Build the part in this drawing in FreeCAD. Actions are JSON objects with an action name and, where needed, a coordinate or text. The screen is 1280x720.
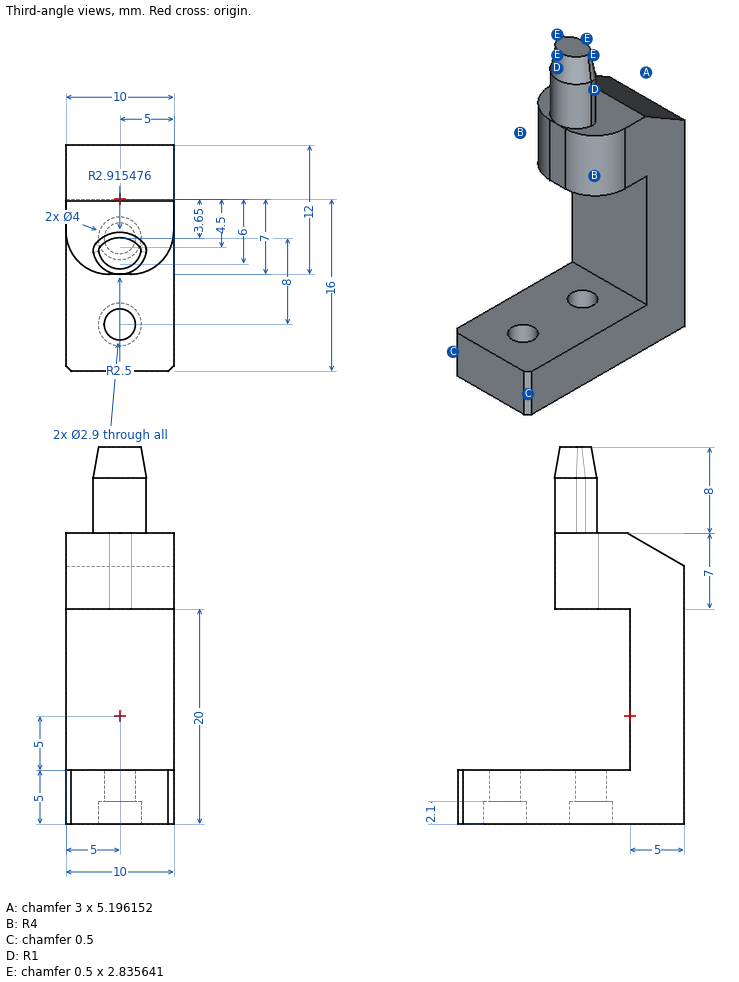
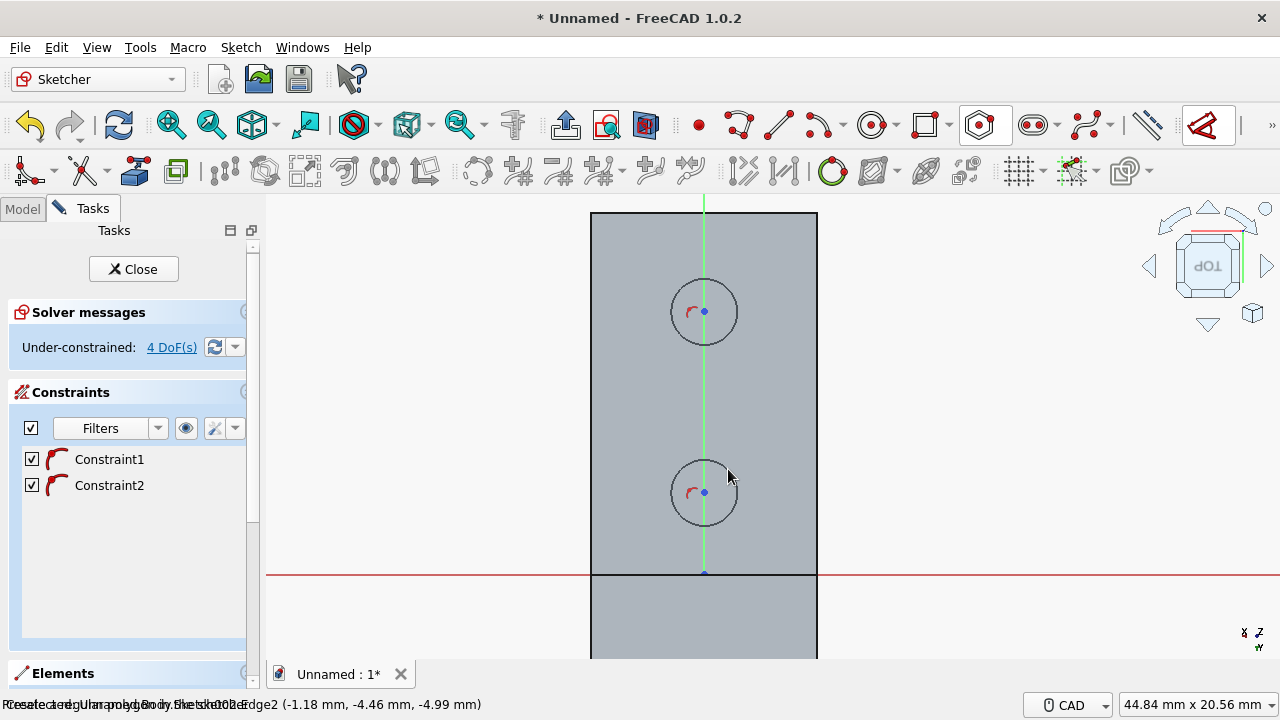
{"action": "left_click", "coordinate": [728, 289]}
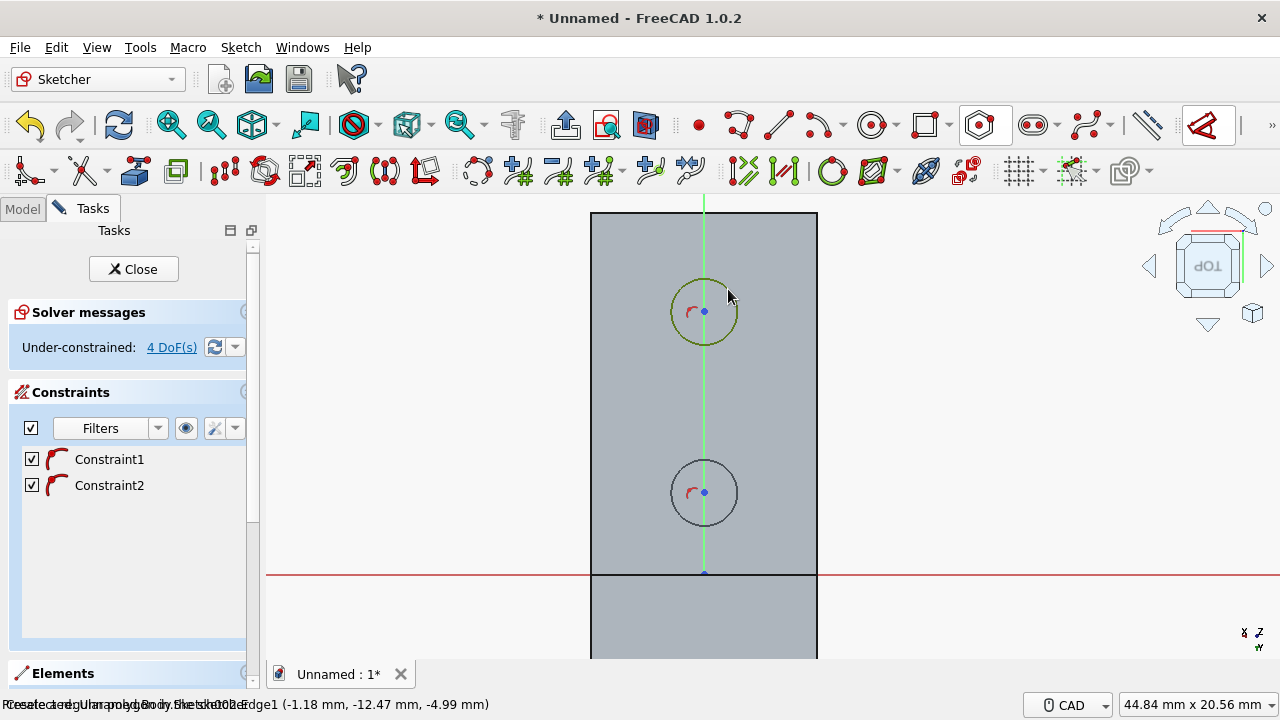
{"action": "left_click", "coordinate": [728, 470]}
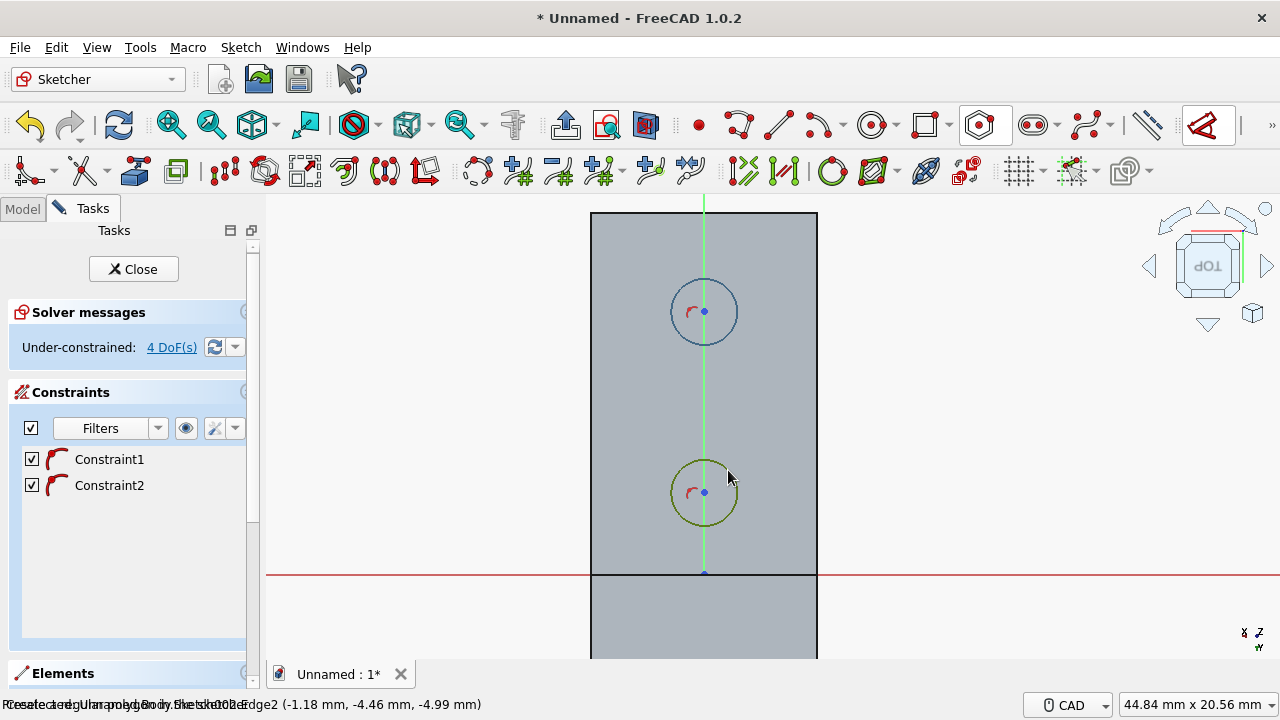
{"action": "key", "text": "e"}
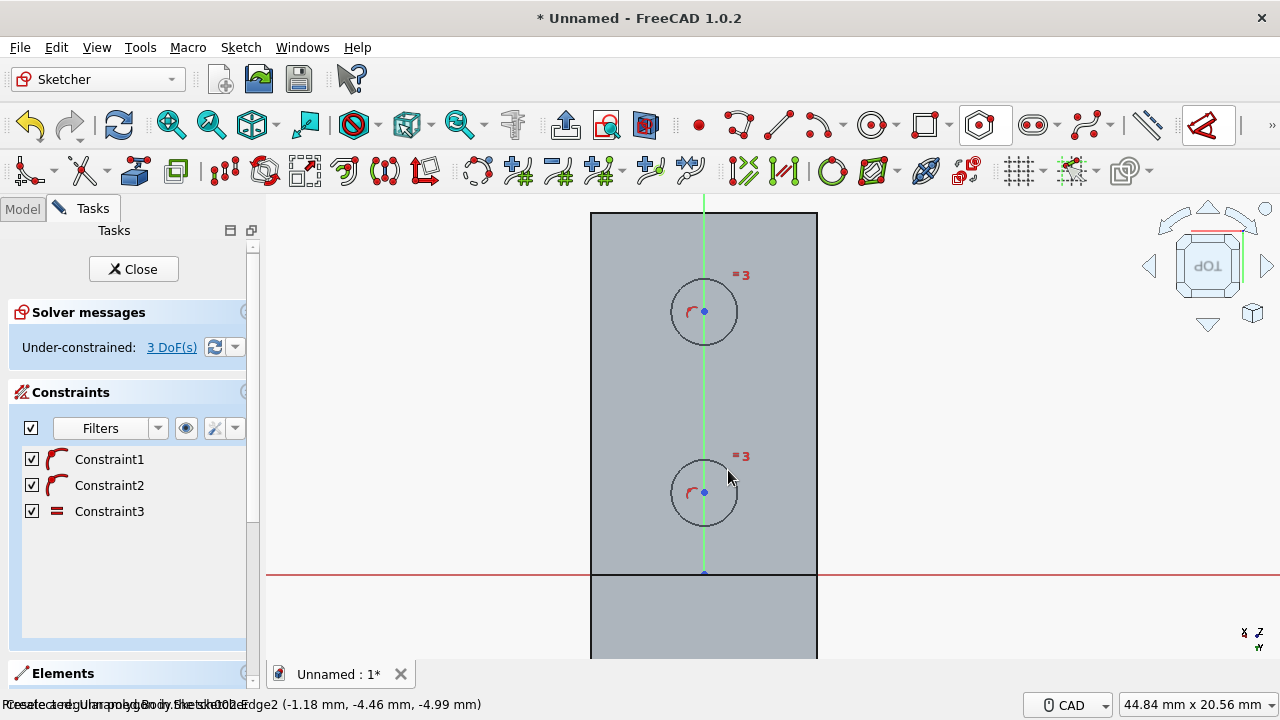
{"action": "key", "text": "d"}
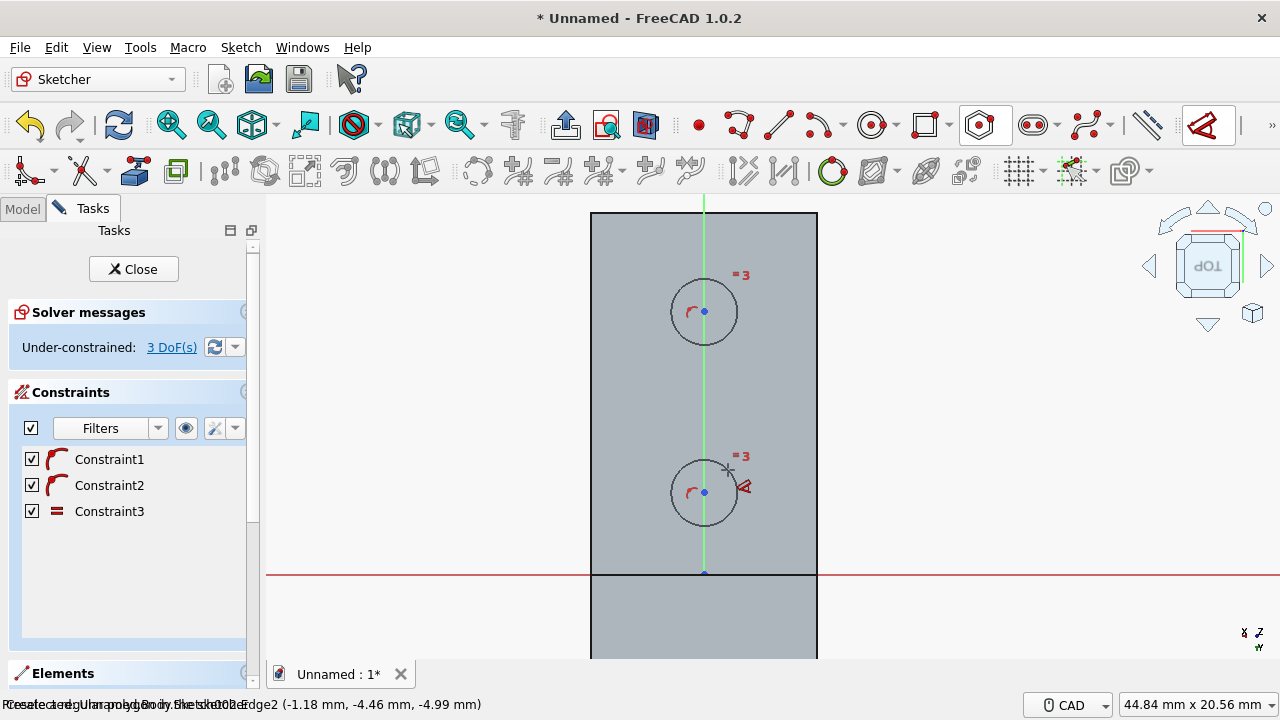
{"action": "left_click", "coordinate": [728, 289]}
{"action": "left_click", "coordinate": [751, 267]}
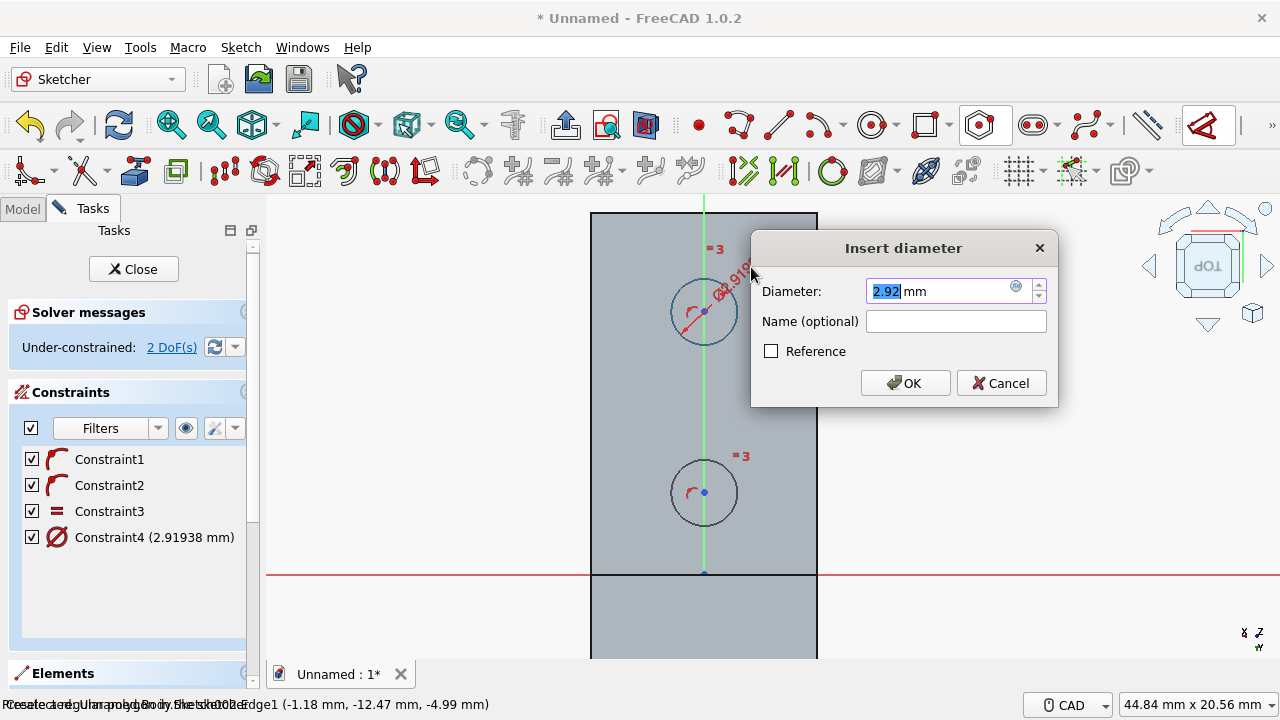
{"action": "type", "text": "2.9"}
{"action": "key", "text": "Return"}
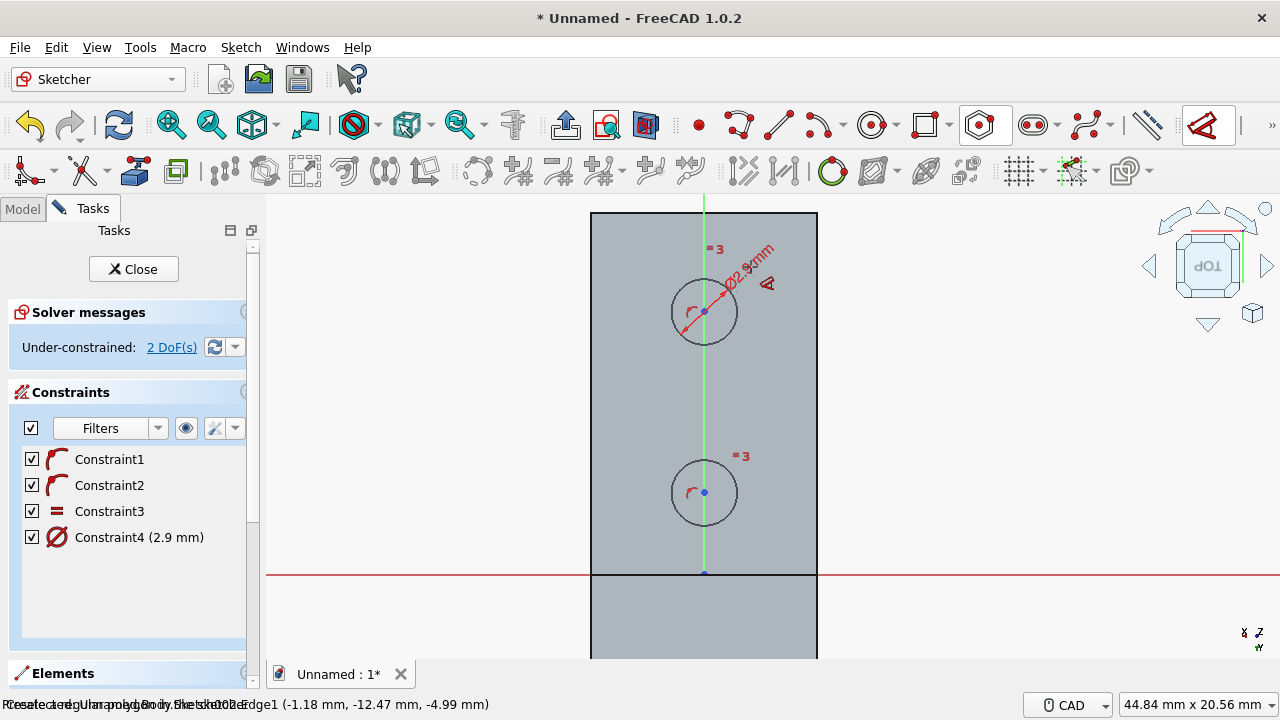
{"action": "left_click", "coordinate": [704, 312]}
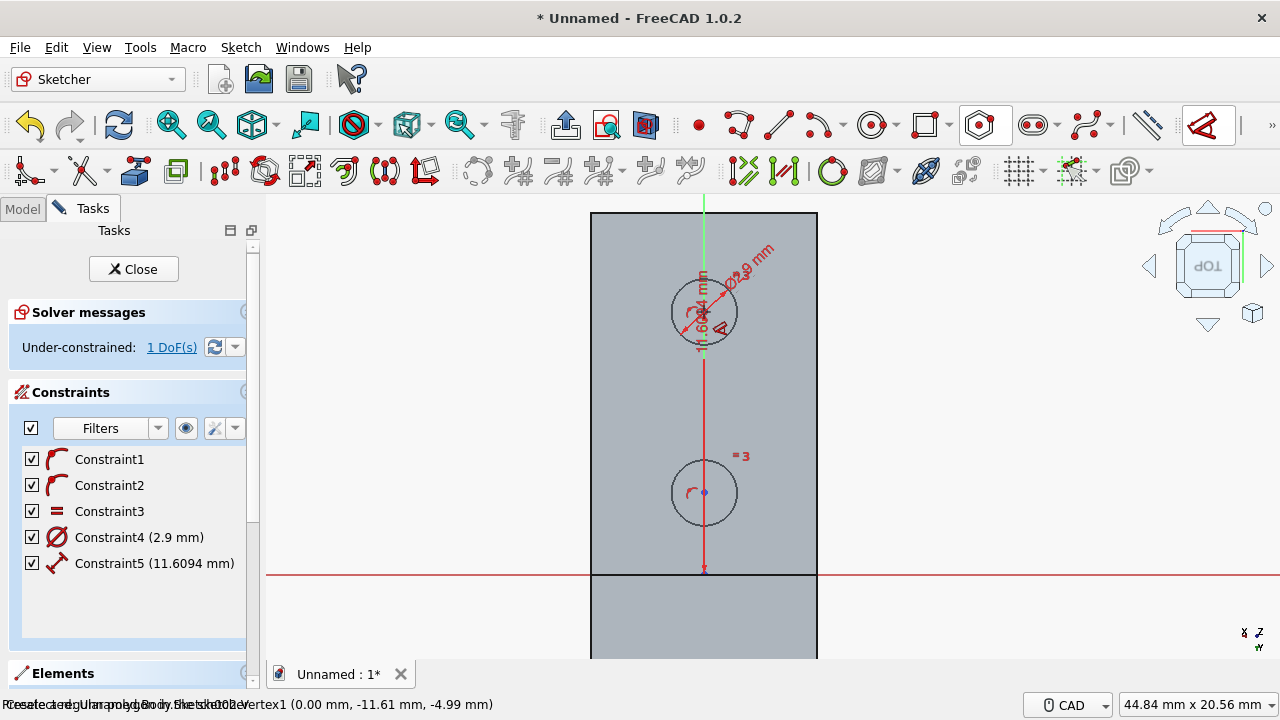
{"action": "left_click", "coordinate": [704, 493]}
{"action": "left_click", "coordinate": [738, 403]}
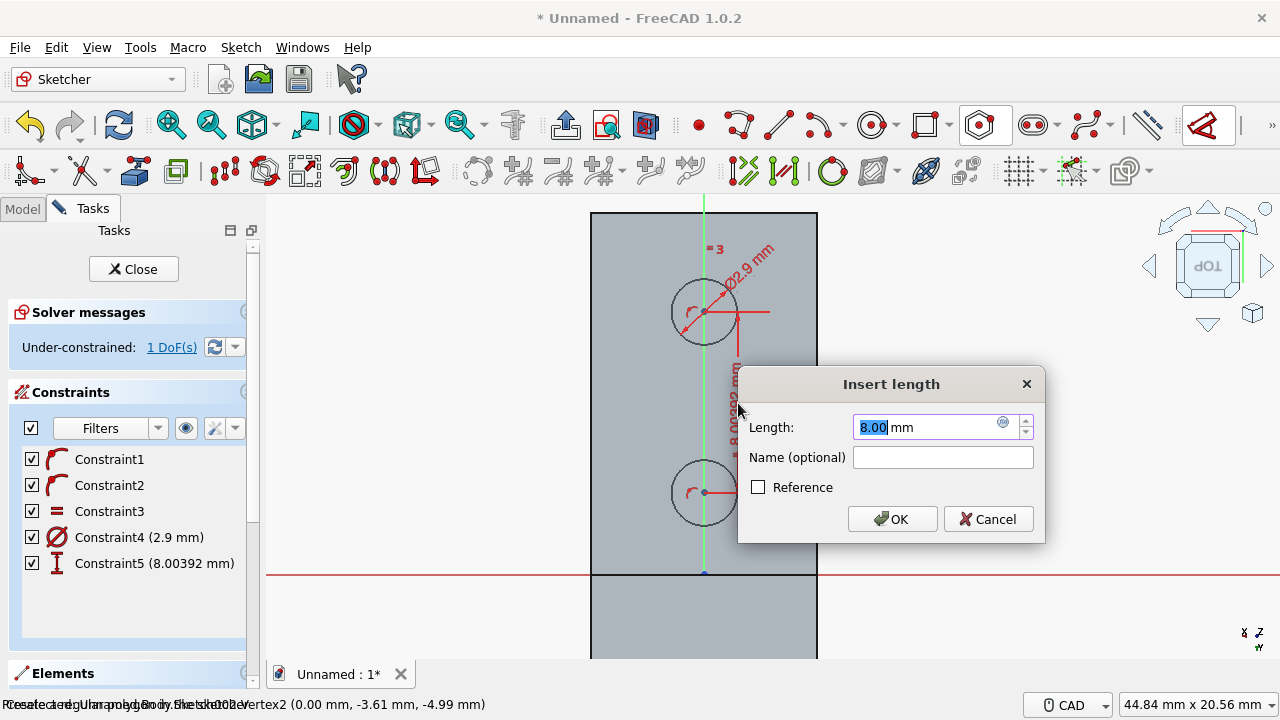
{"action": "type", "text": "8"}
{"action": "key", "text": "Return"}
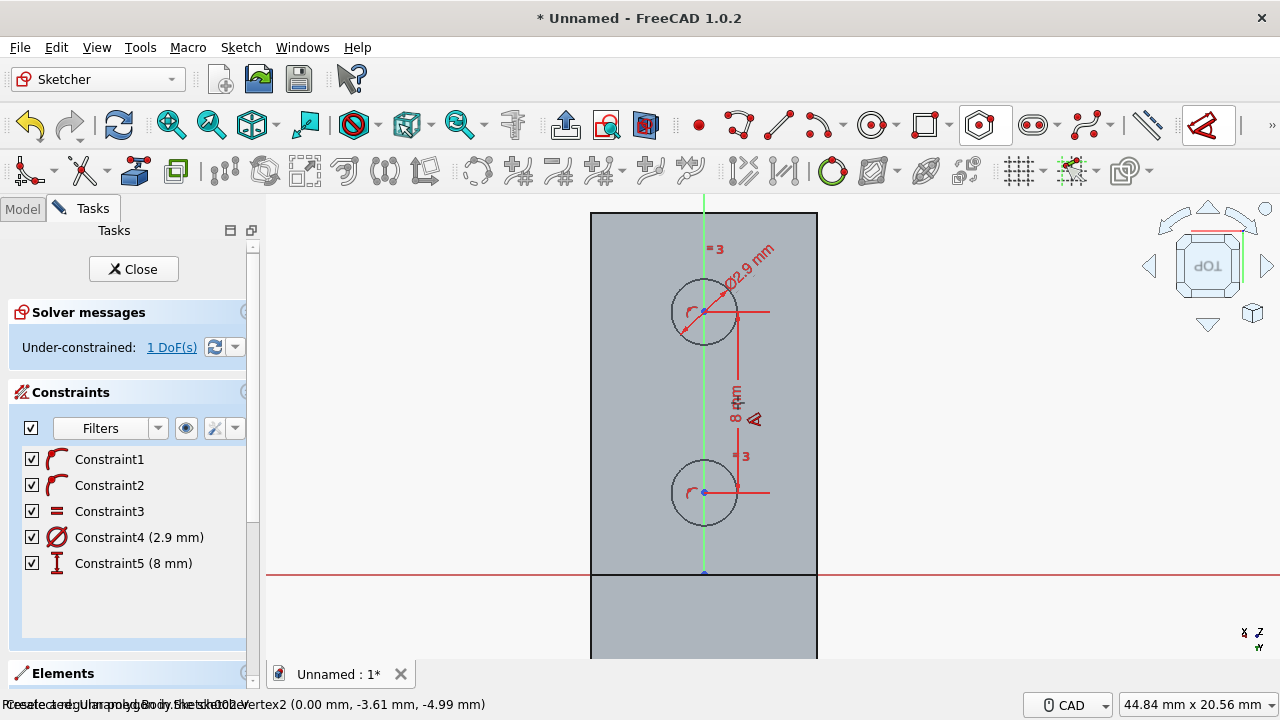
{"action": "left_click", "coordinate": [704, 493]}
{"action": "left_click", "coordinate": [738, 534]}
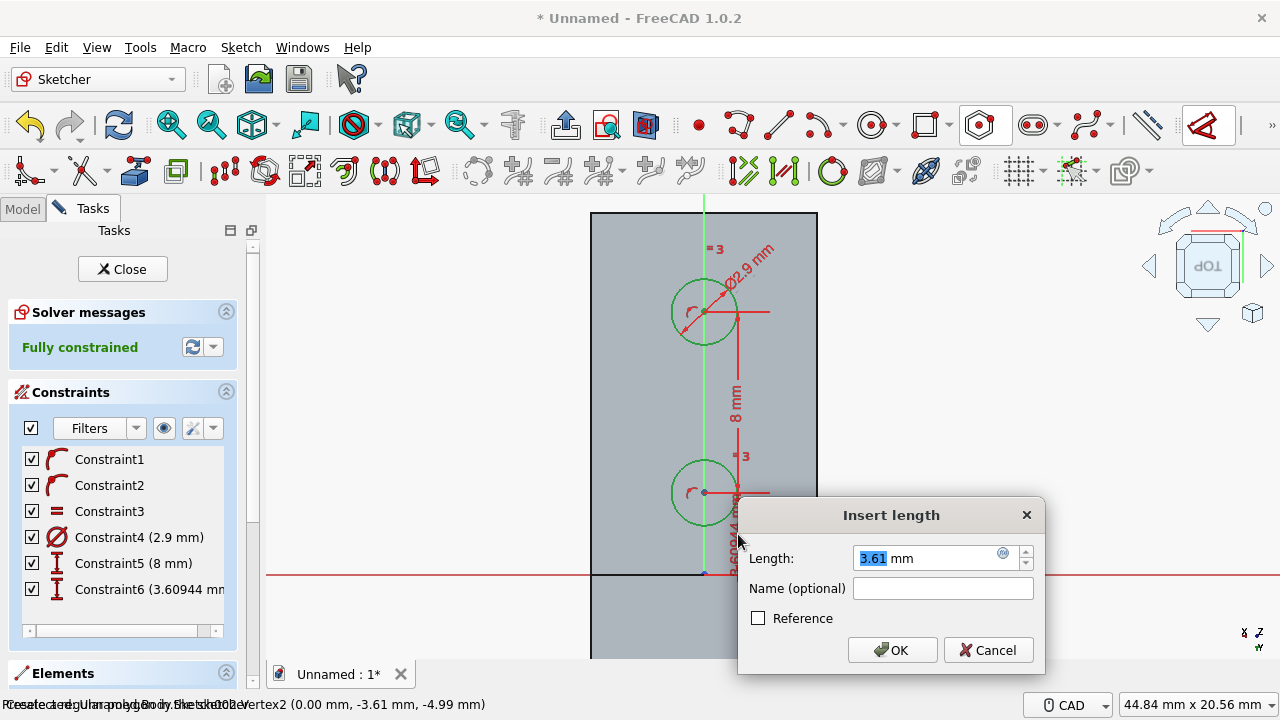
{"action": "type", "text": "3.65"}
{"action": "key", "text": "Return"}
{"action": "key", "text": "Escape"}